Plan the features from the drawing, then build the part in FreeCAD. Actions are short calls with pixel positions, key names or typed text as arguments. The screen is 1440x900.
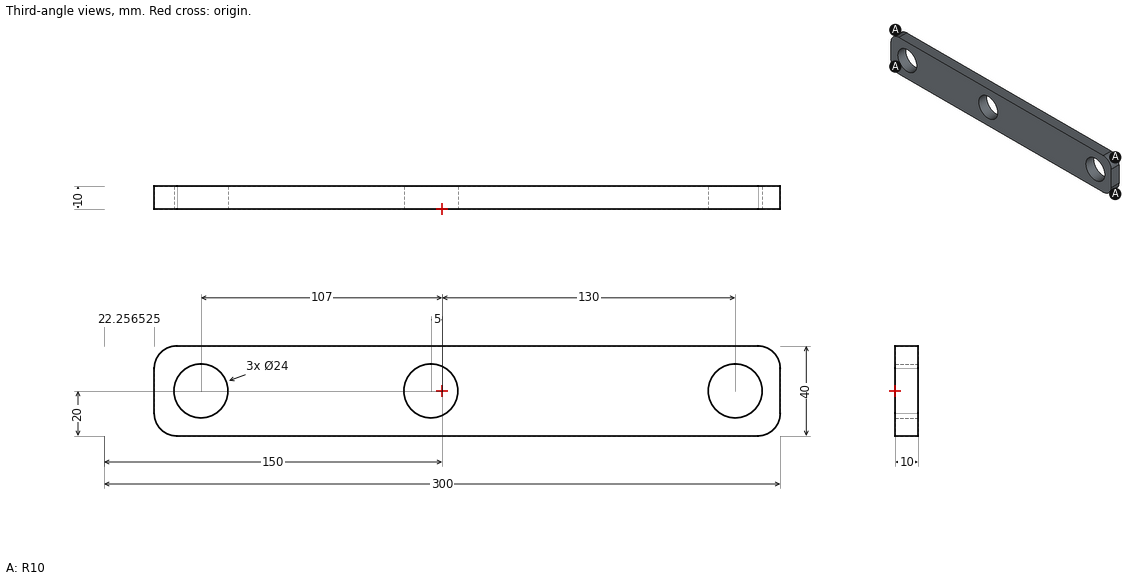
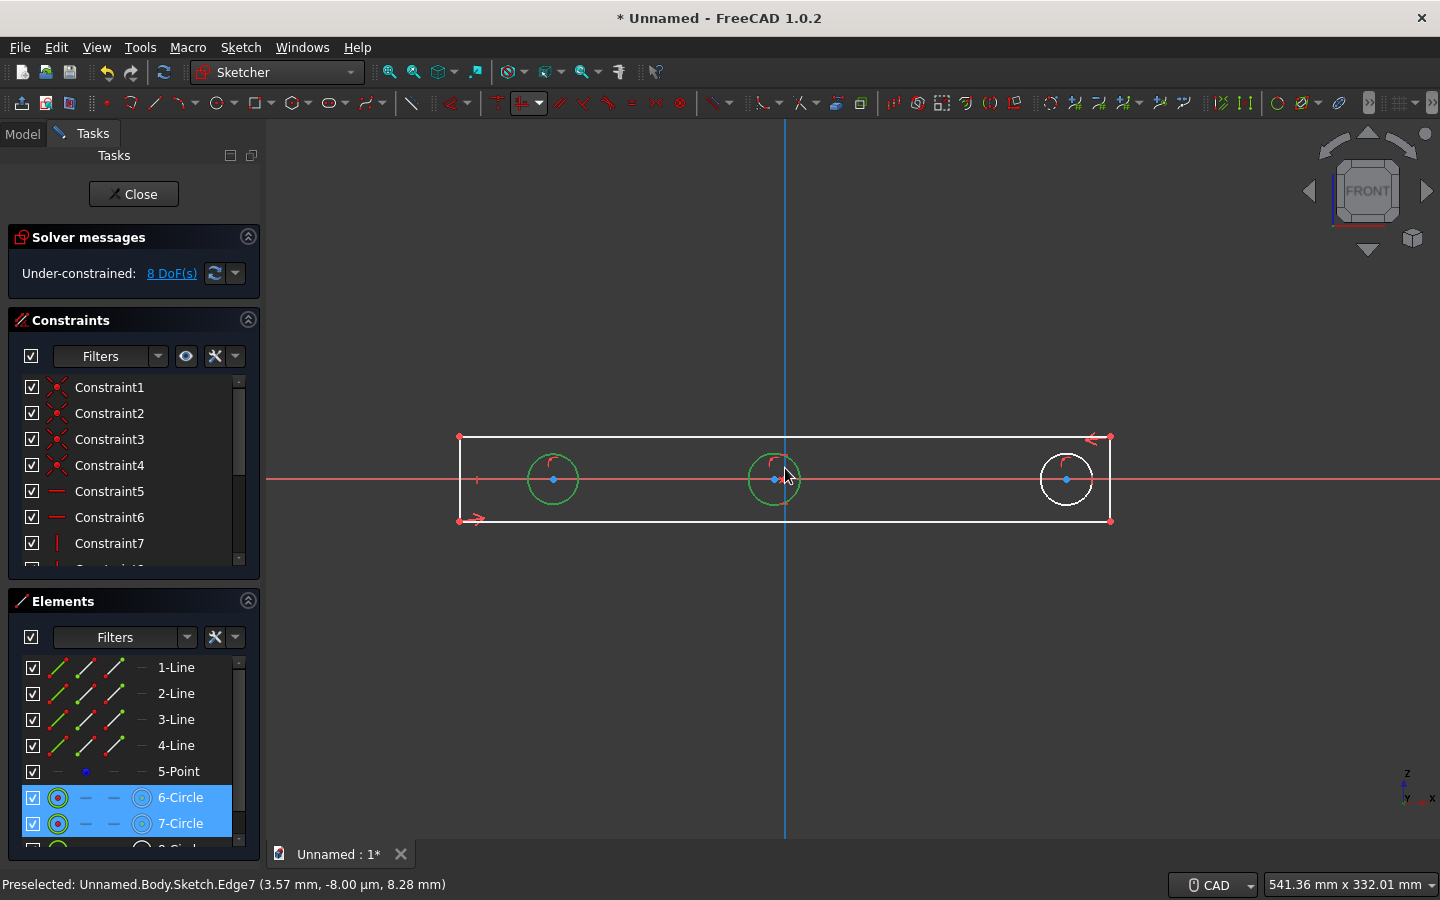
click(1085, 461)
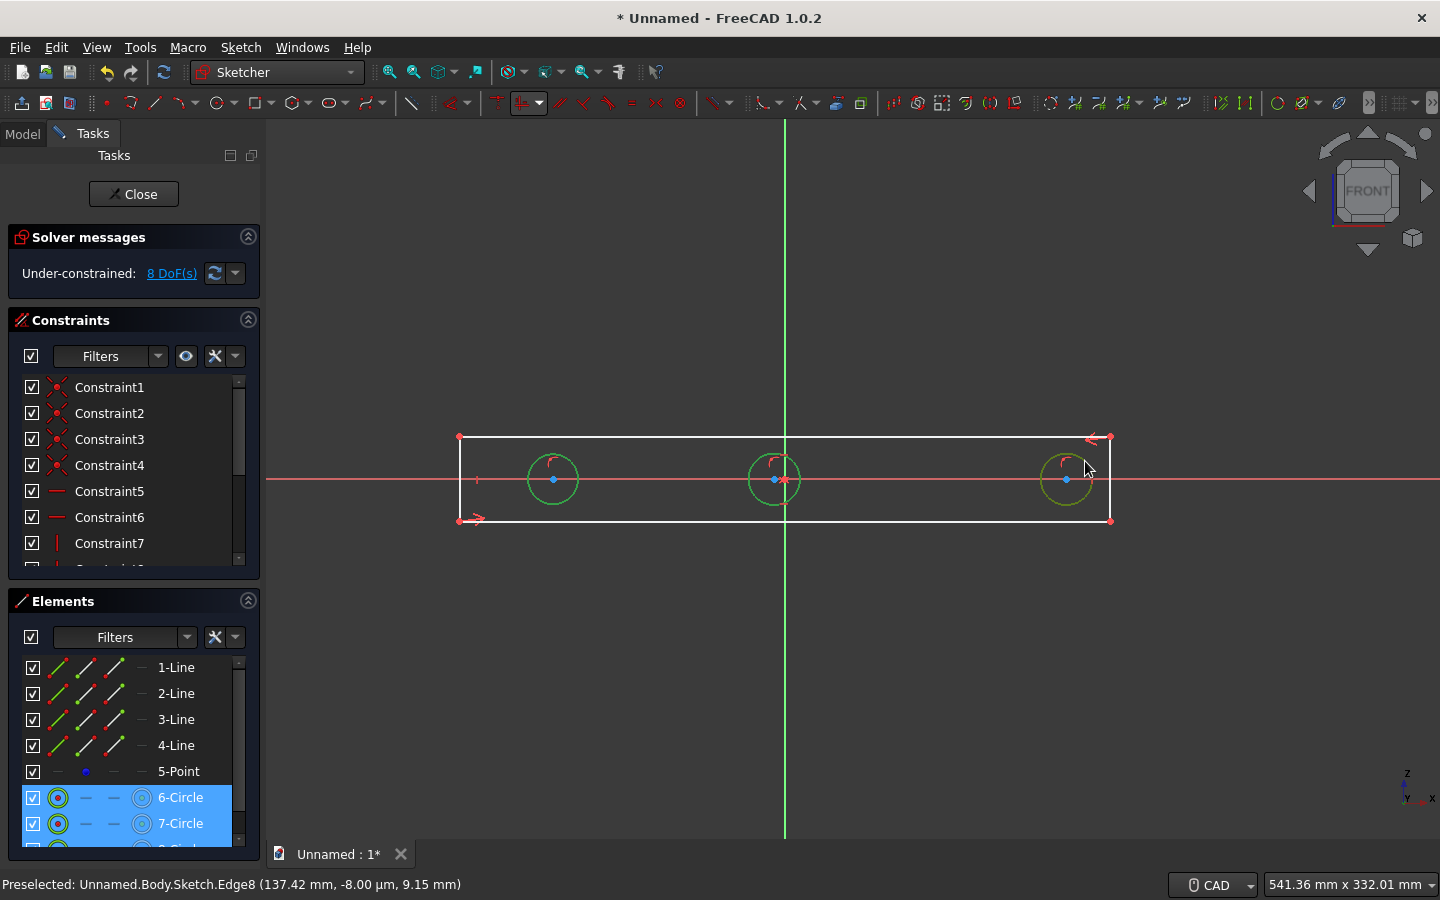
click(632, 104)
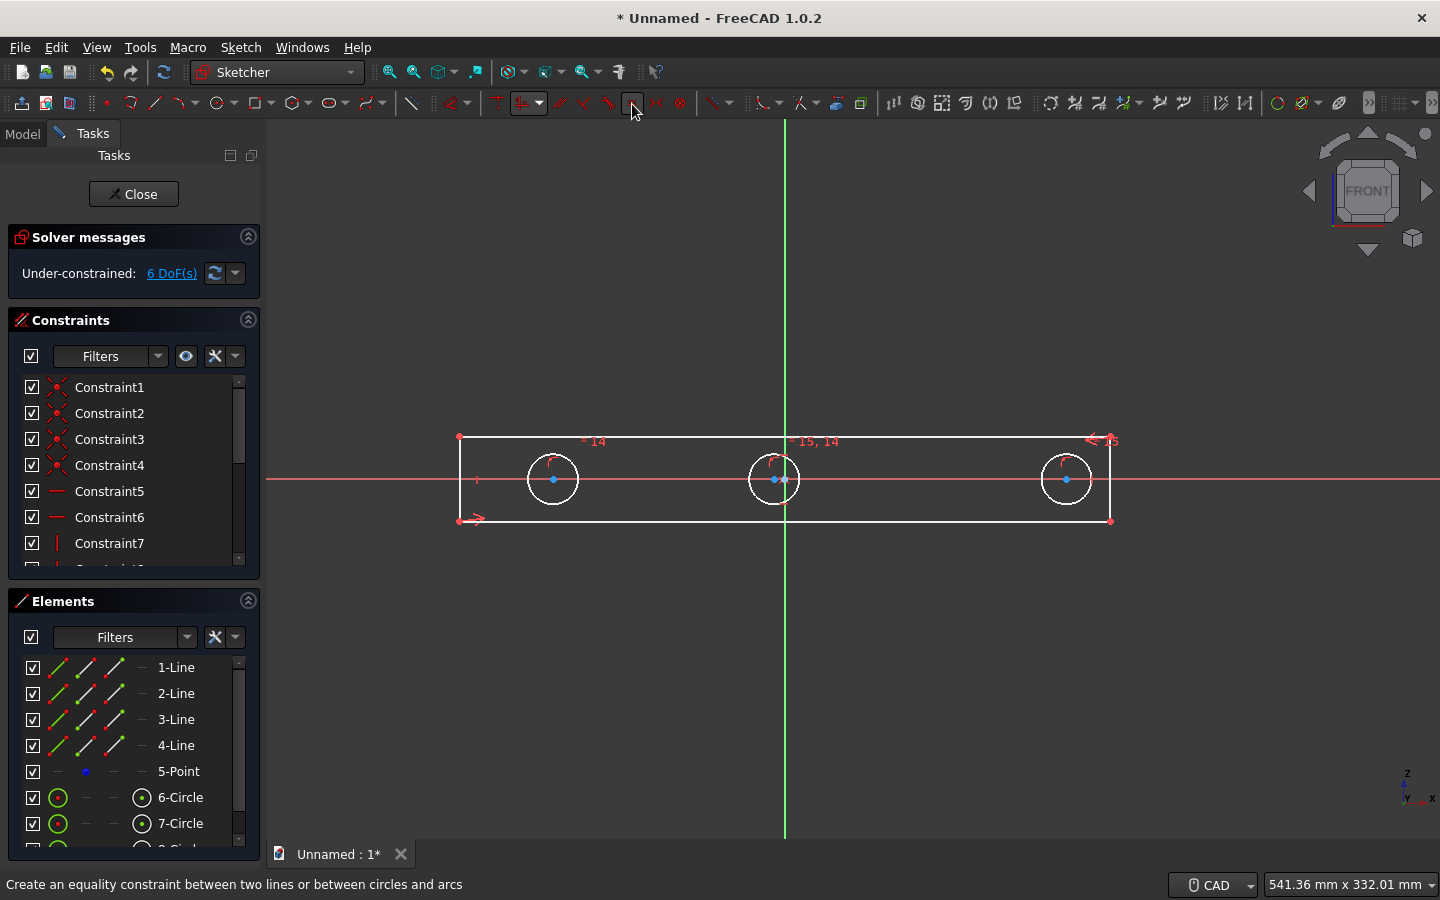
click(571, 462)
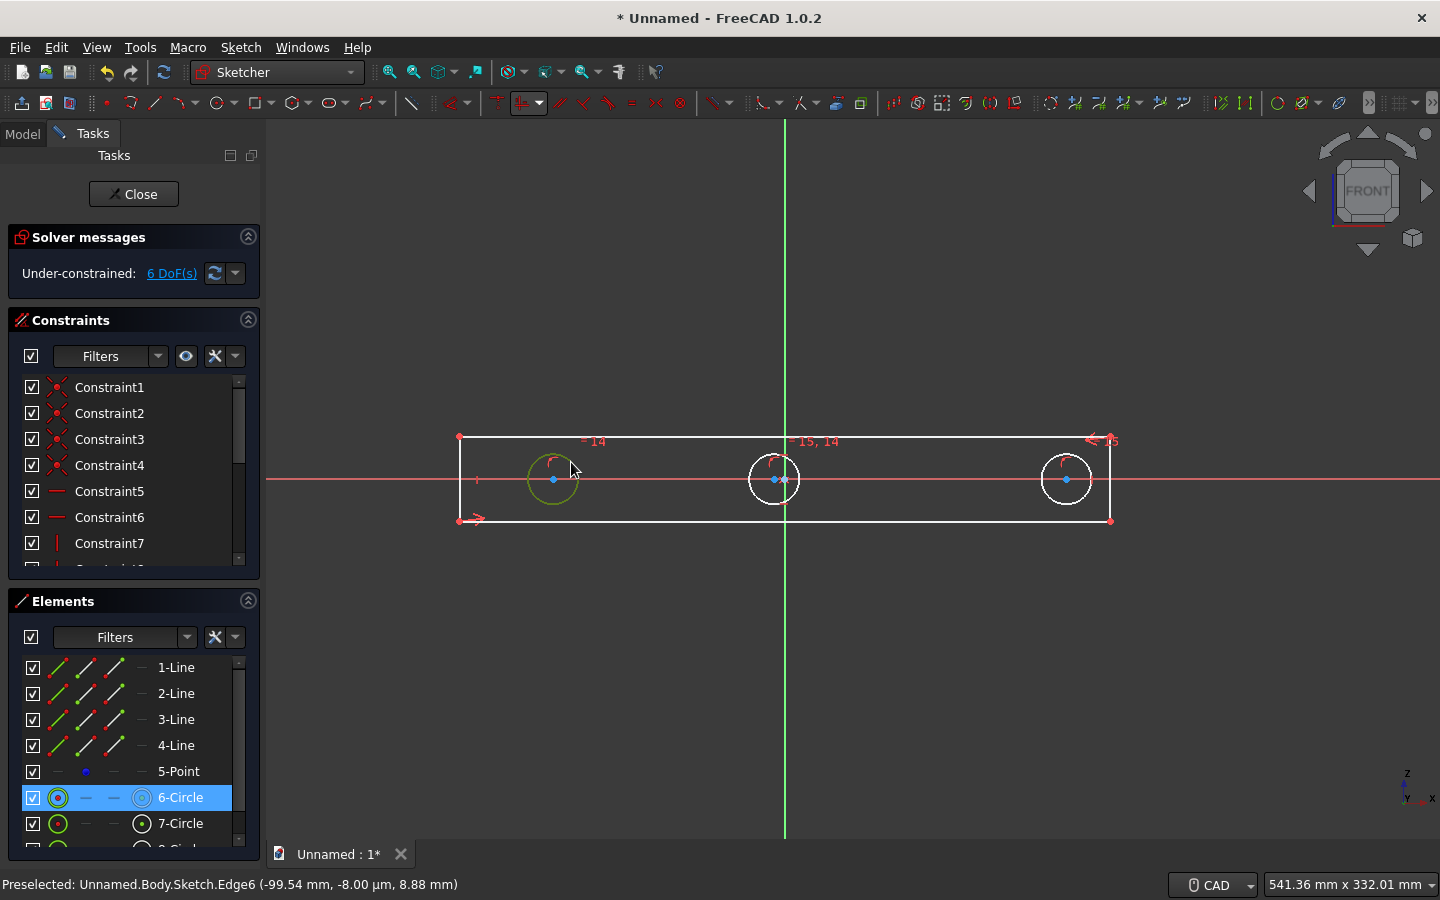
click(470, 104)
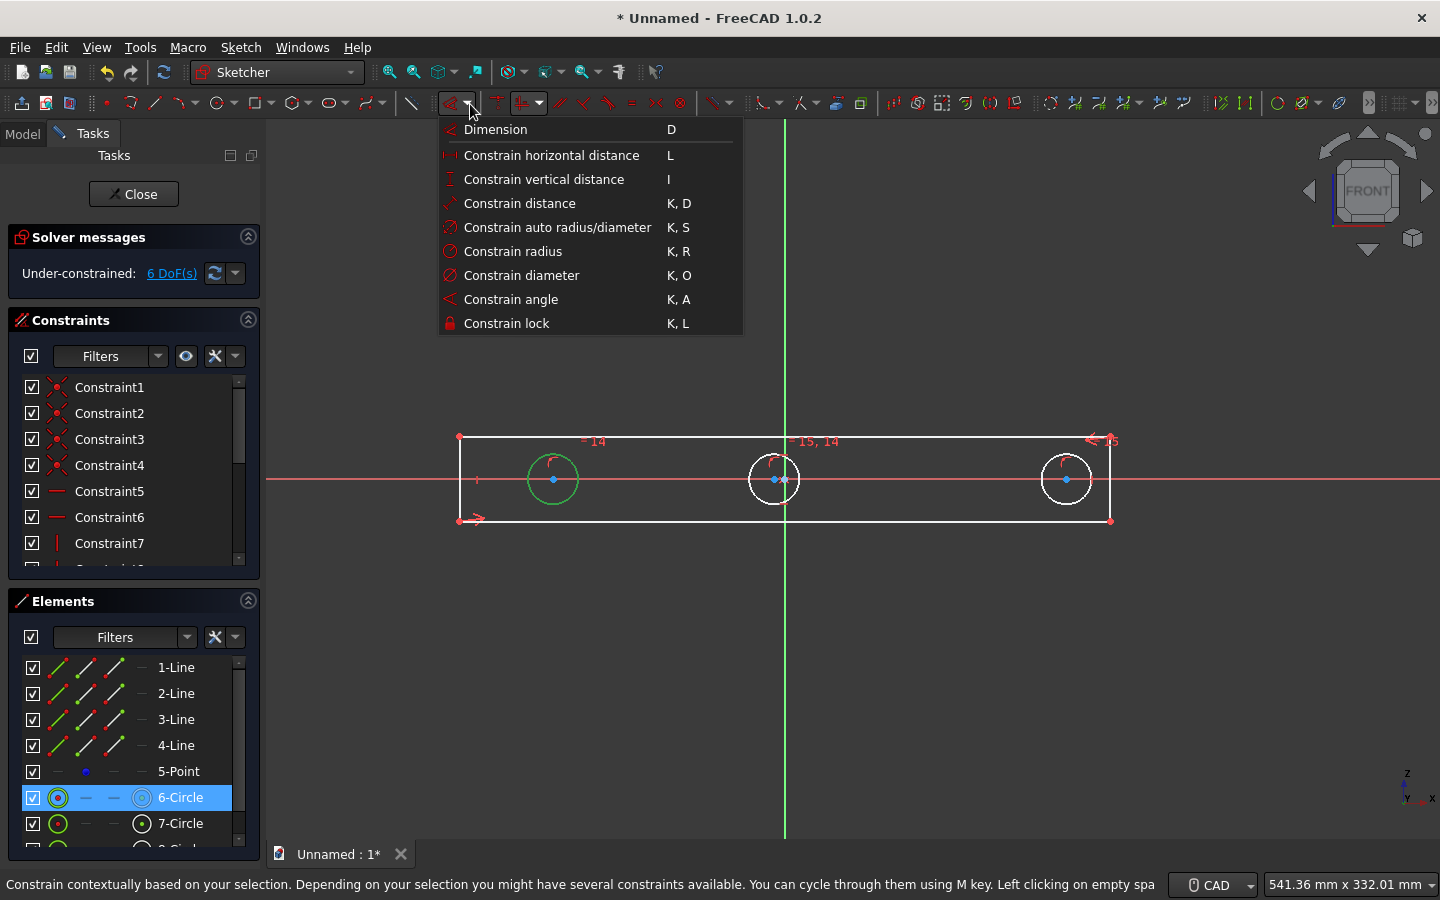
click(591, 275)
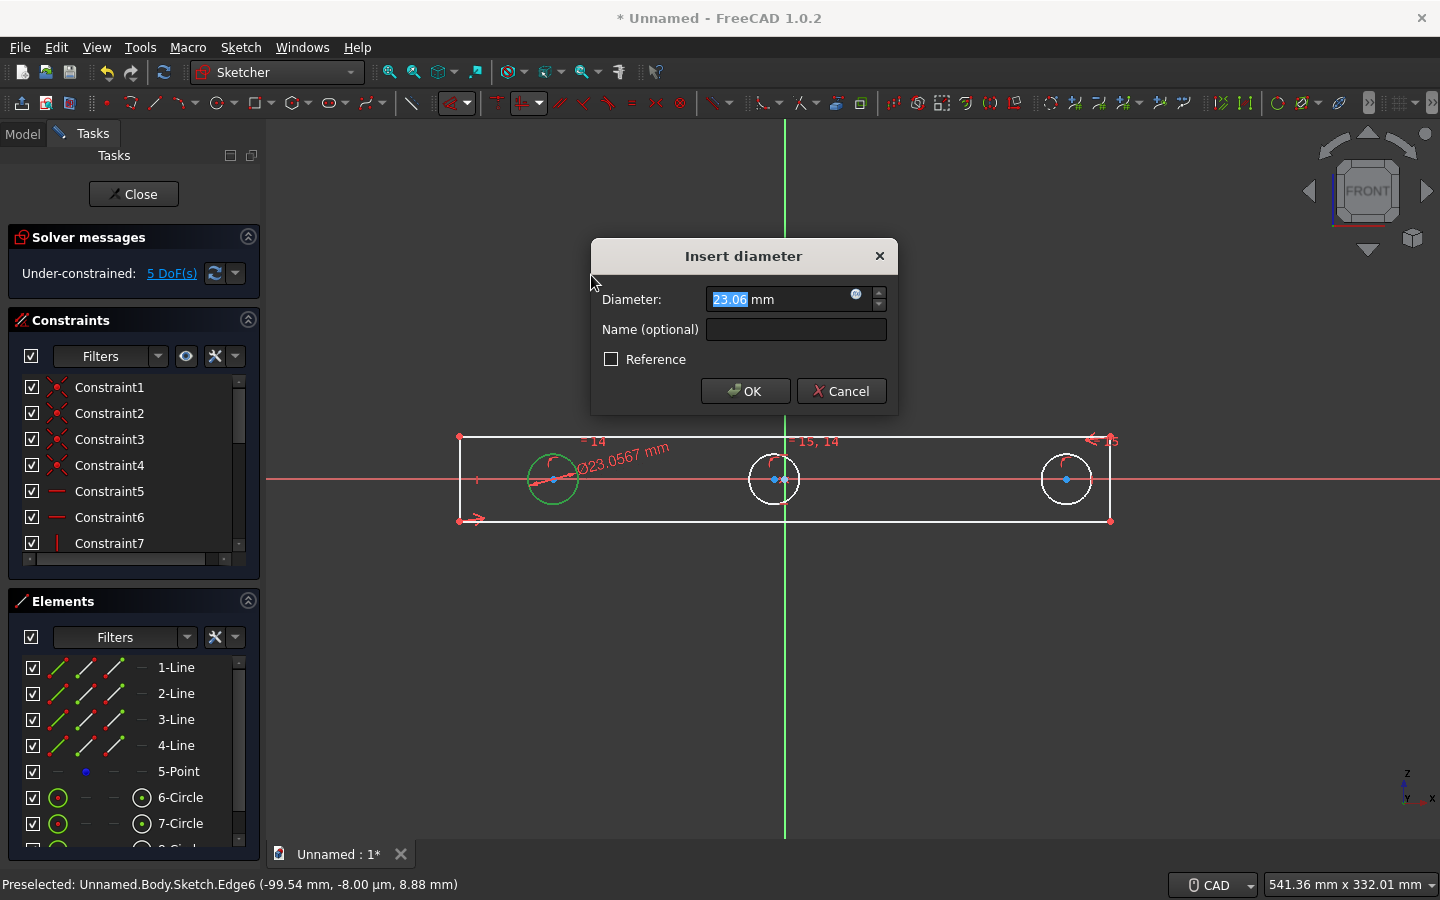
text(24)
key(Return)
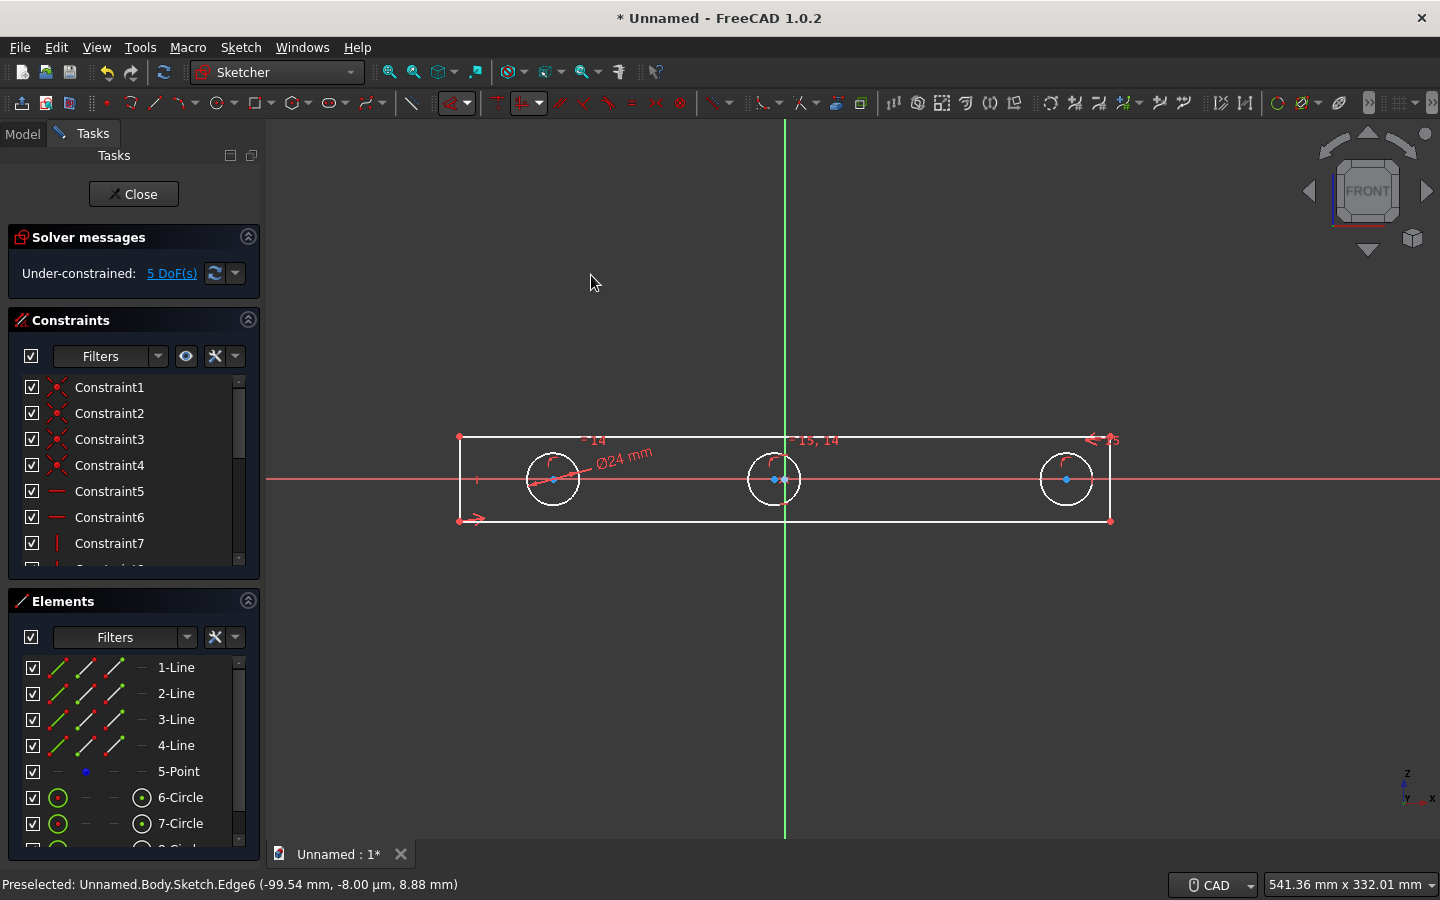
scroll(774, 479, up, 7)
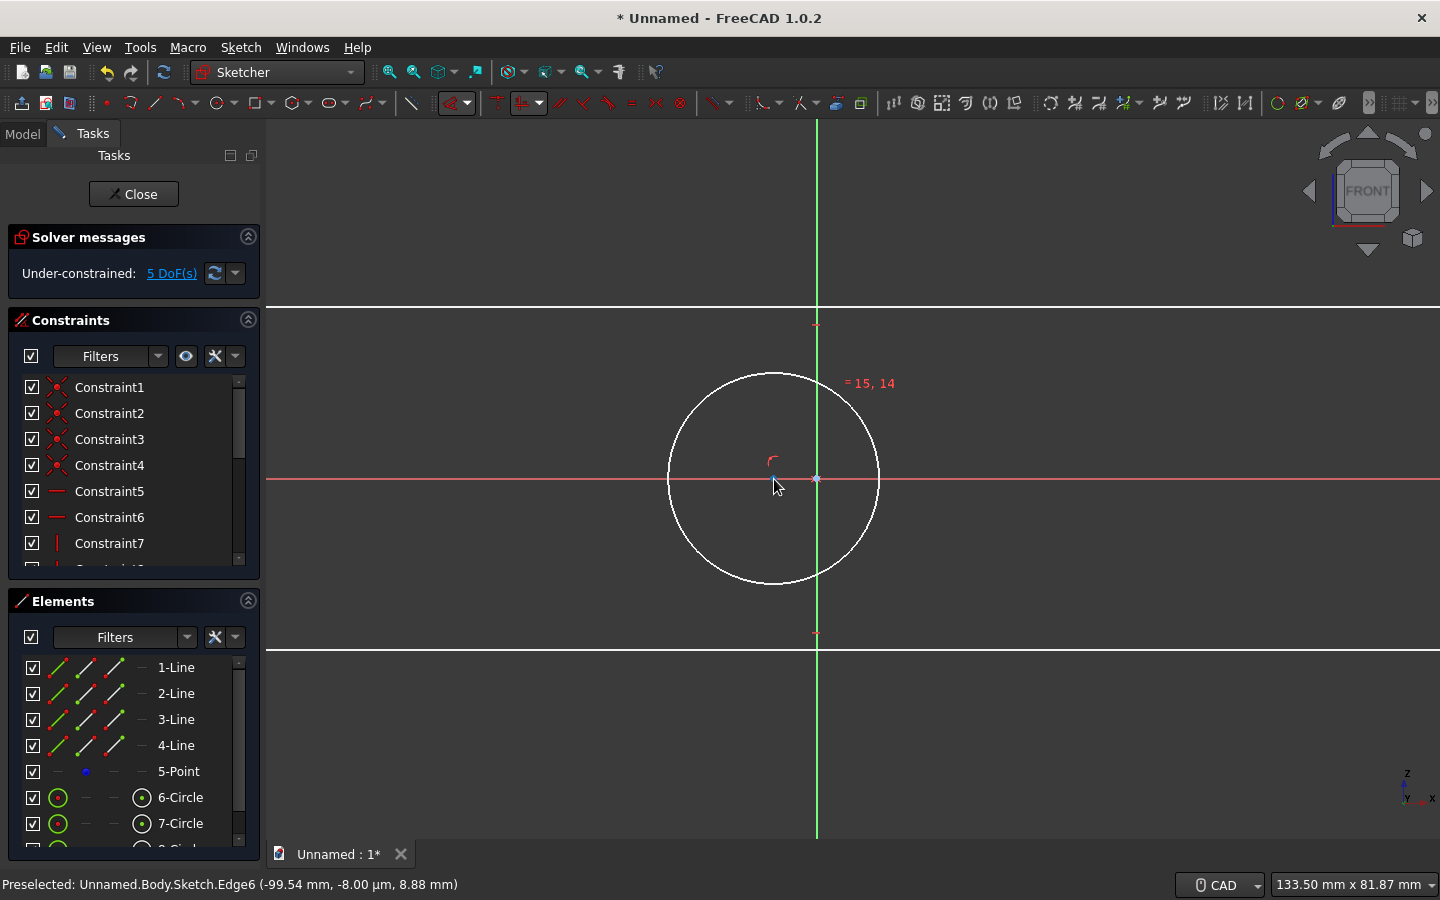
click(774, 479)